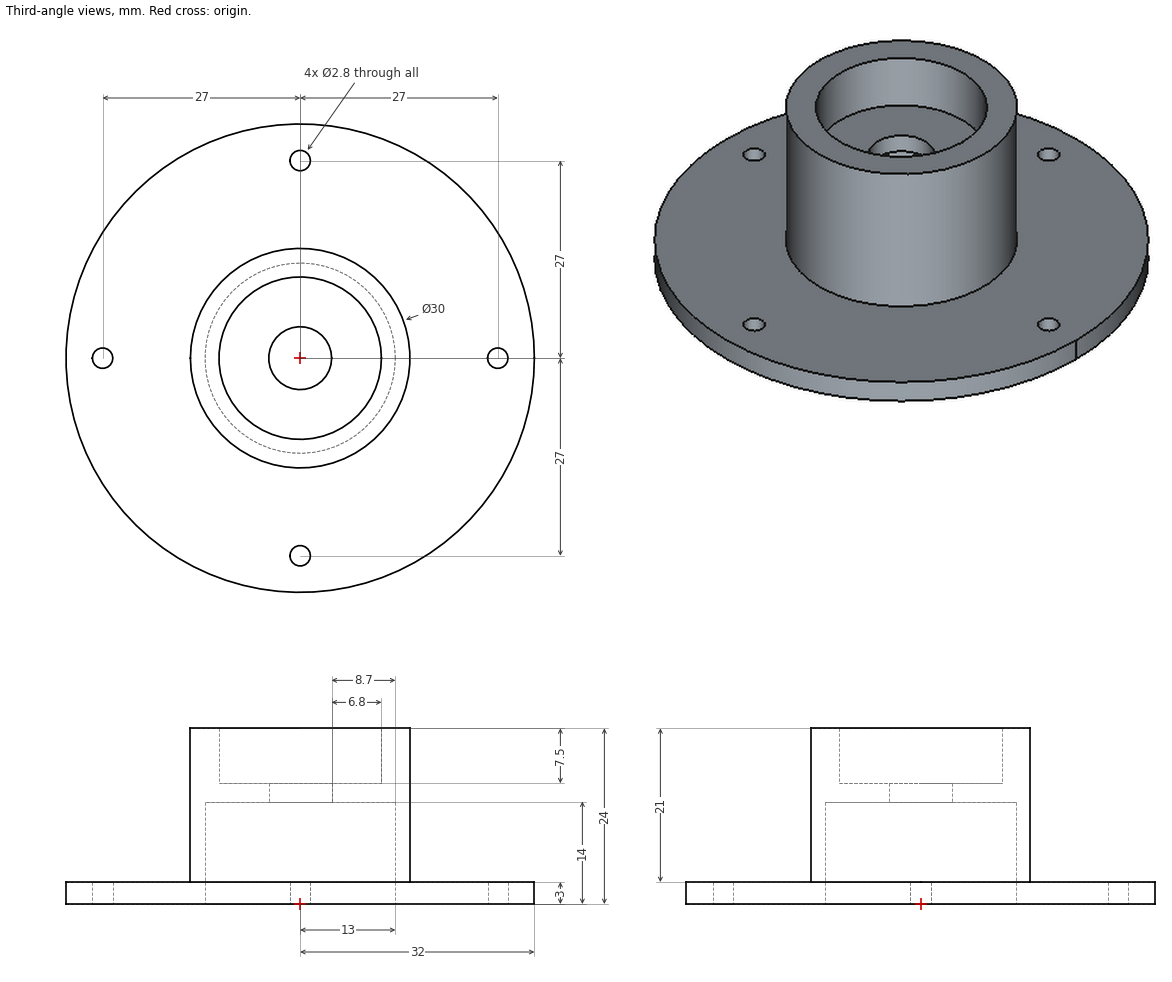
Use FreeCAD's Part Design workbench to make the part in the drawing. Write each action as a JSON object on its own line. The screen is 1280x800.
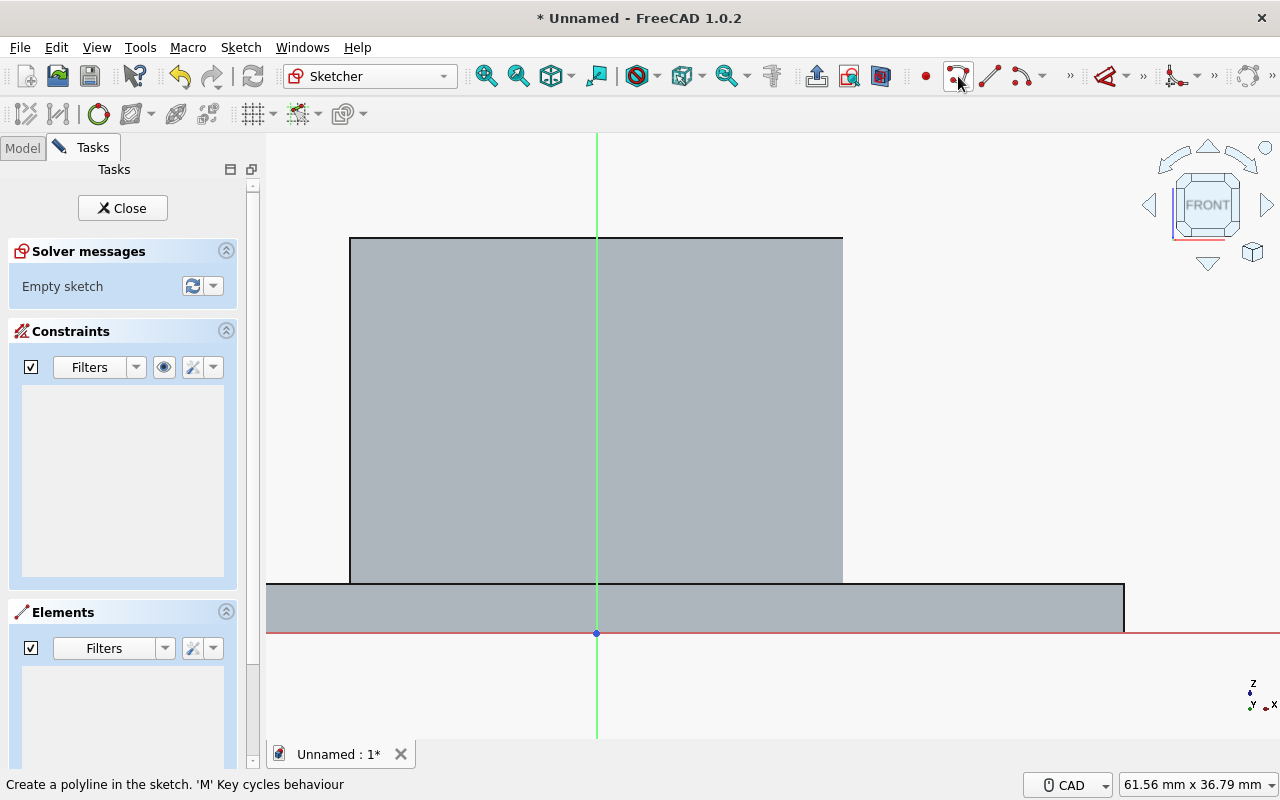
{"action": "left_click", "coordinate": [597, 633]}
{"action": "left_click", "coordinate": [606, 238]}
{"action": "left_click", "coordinate": [780, 238]}
{"action": "left_click", "coordinate": [780, 361]}
{"action": "left_click", "coordinate": [668, 361]}
{"action": "left_click", "coordinate": [668, 402]}
{"action": "left_click", "coordinate": [811, 402]}
{"action": "left_click", "coordinate": [811, 624]}
{"action": "left_click", "coordinate": [597, 633]}
{"action": "key", "text": "Escape"}
{"action": "key", "text": "Escape"}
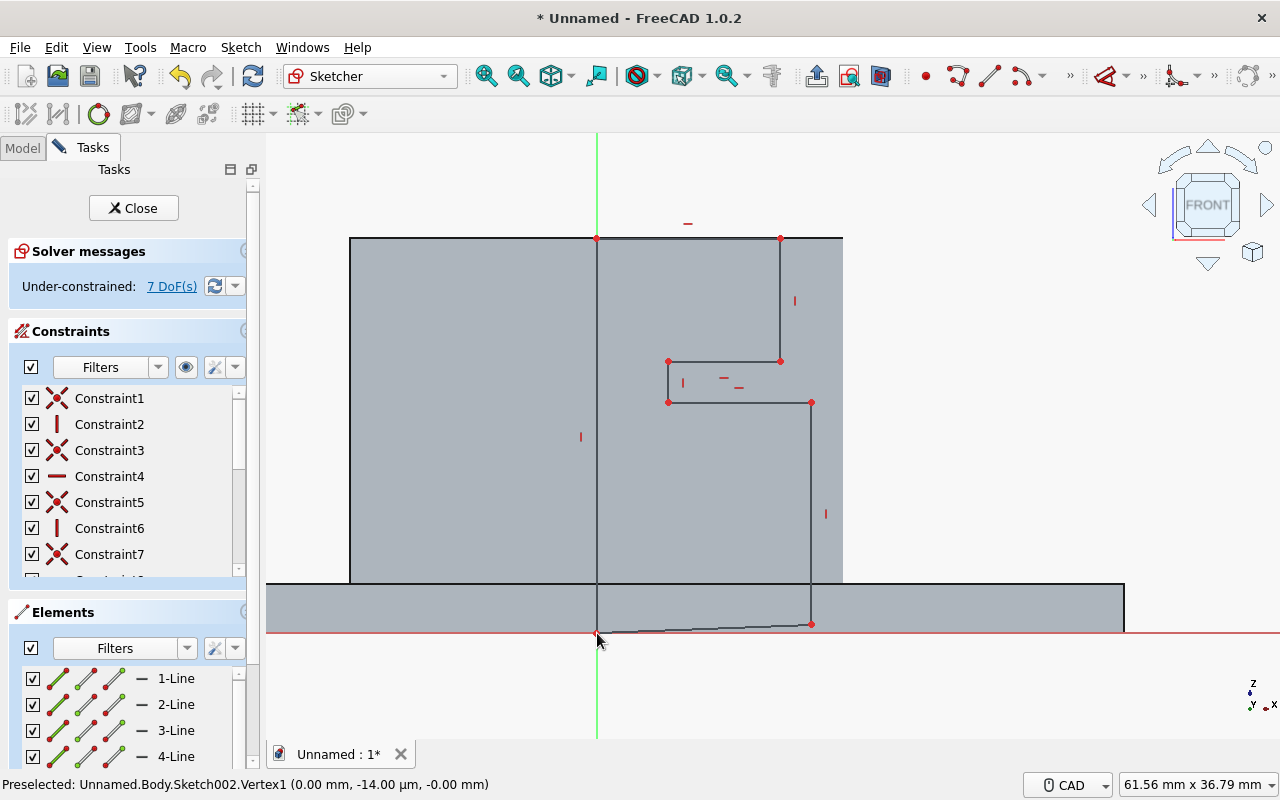
{"action": "left_click", "coordinate": [661, 631]}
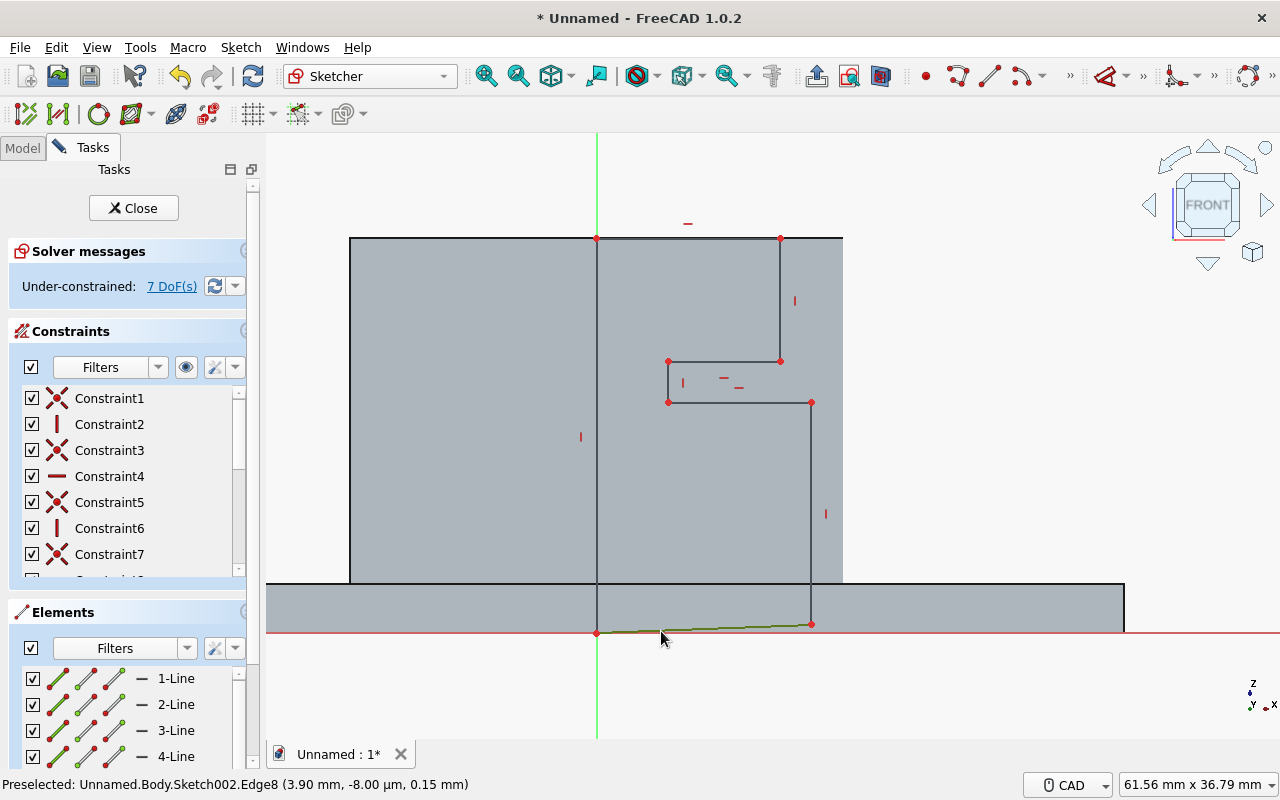
{"action": "key", "text": "h"}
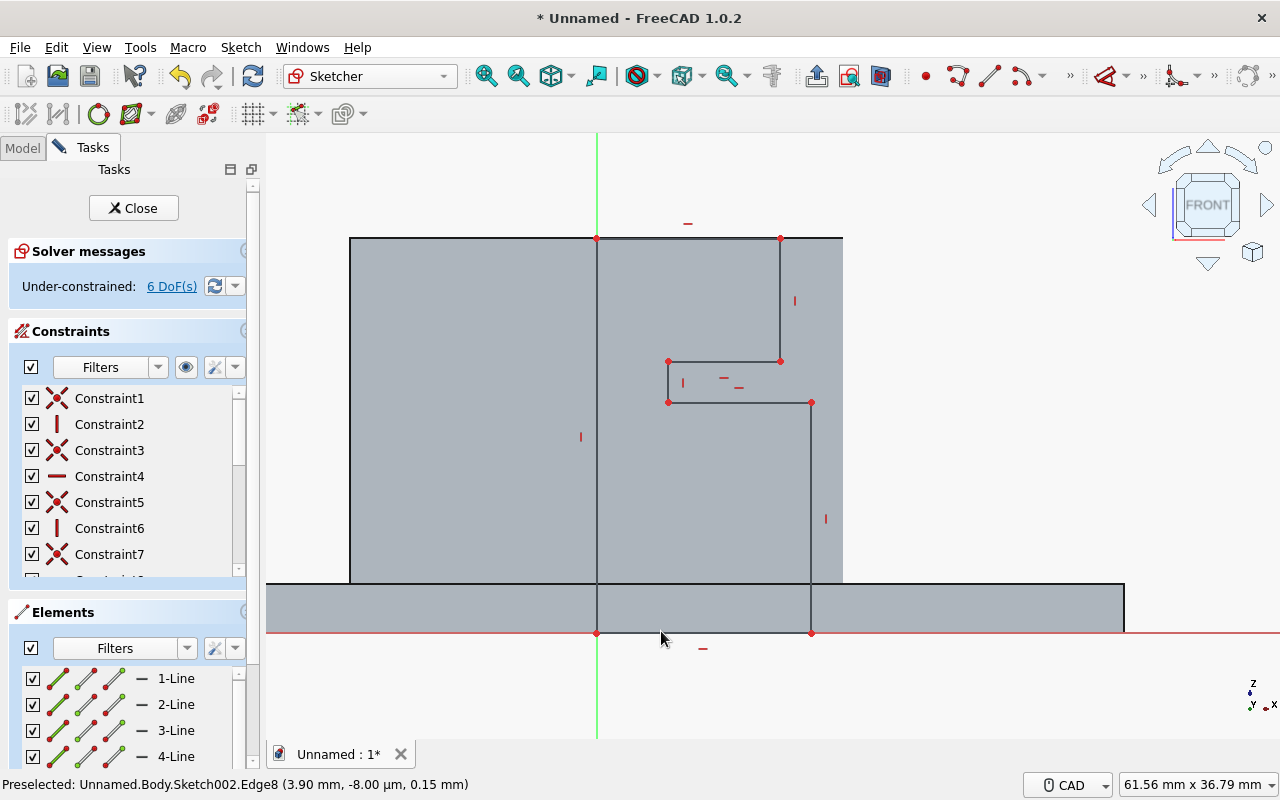
{"action": "key", "text": "d"}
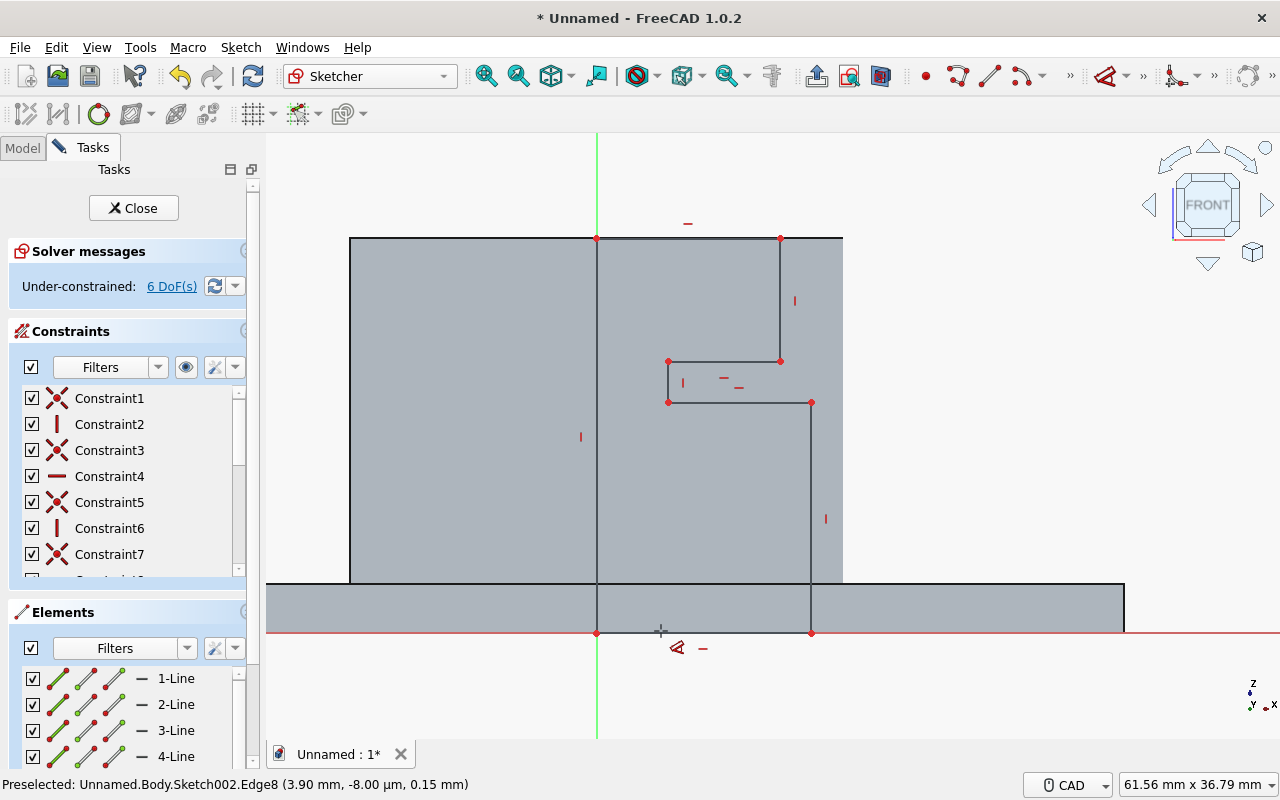
{"action": "left_click", "coordinate": [597, 515]}
{"action": "left_click", "coordinate": [563, 436]}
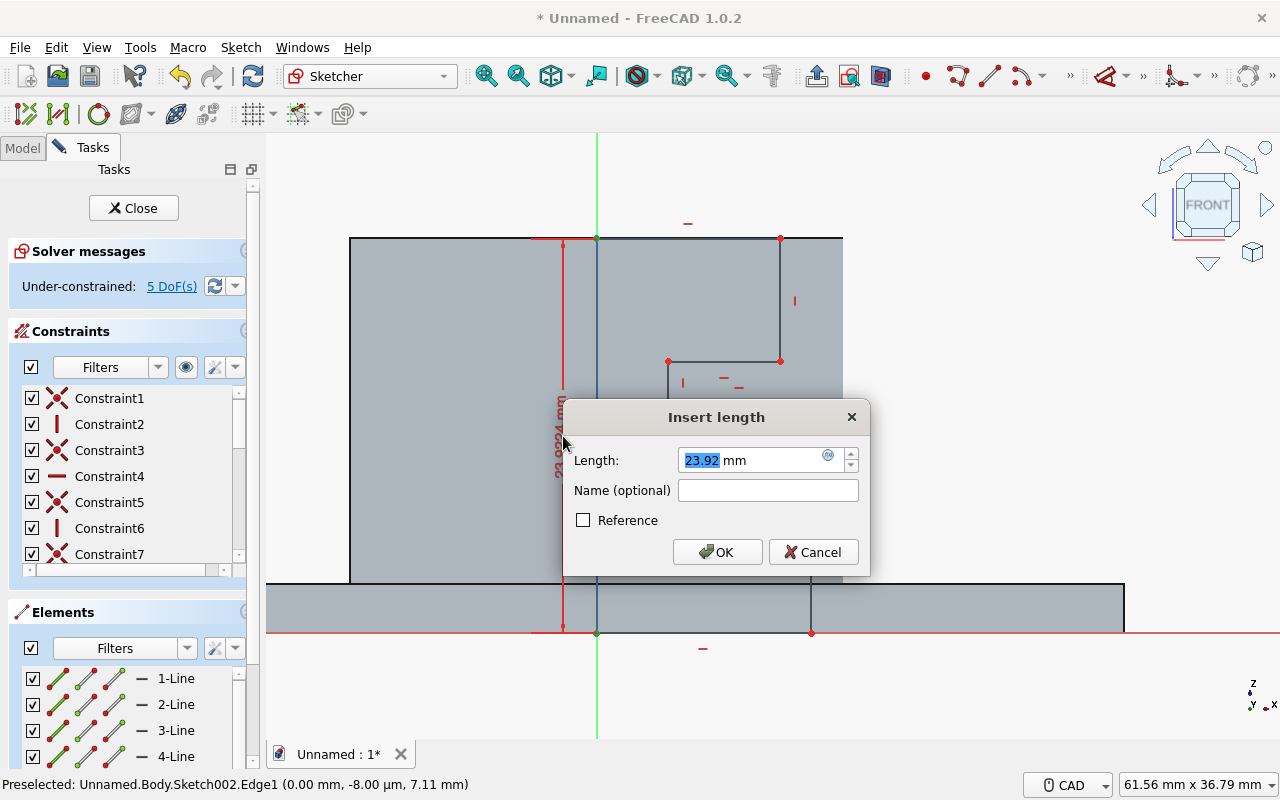
{"action": "type", "text": "24"}
{"action": "key", "text": "Return"}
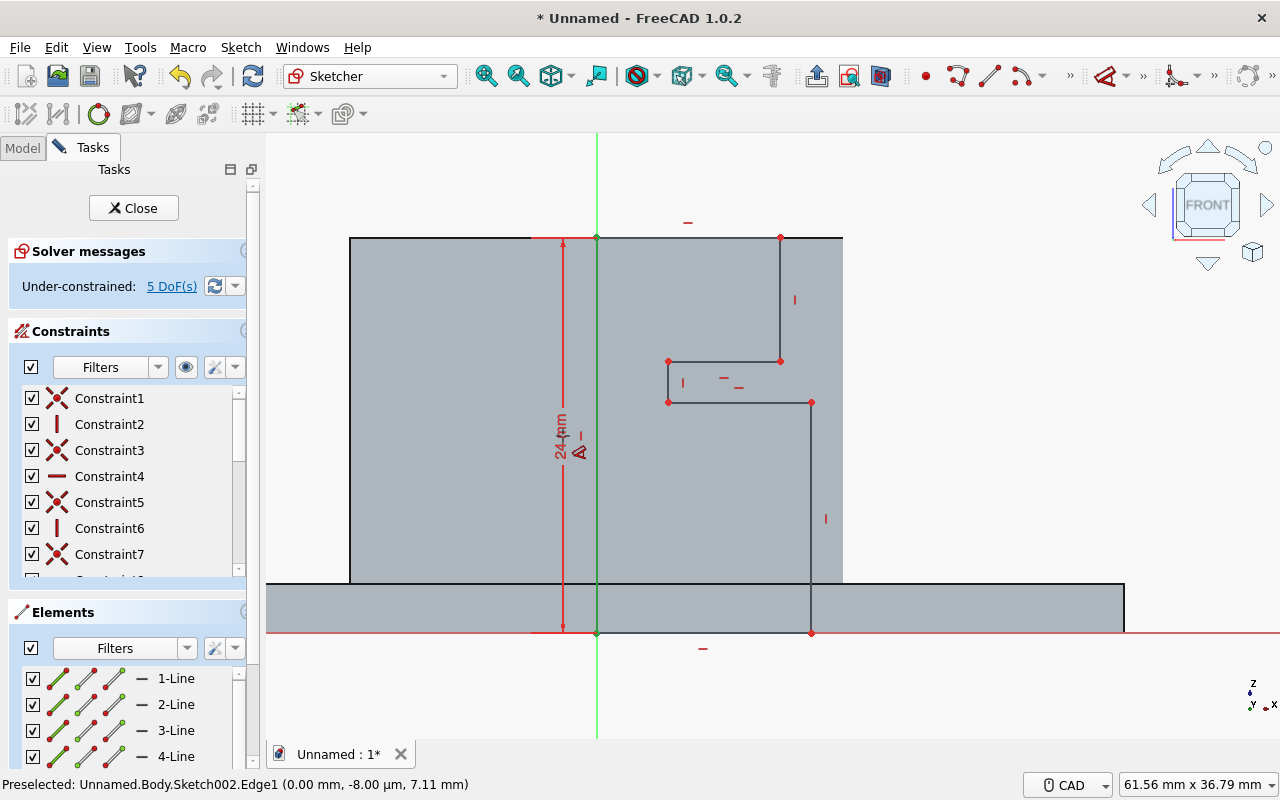
{"action": "left_click", "coordinate": [811, 472]}
{"action": "left_click", "coordinate": [845, 518]}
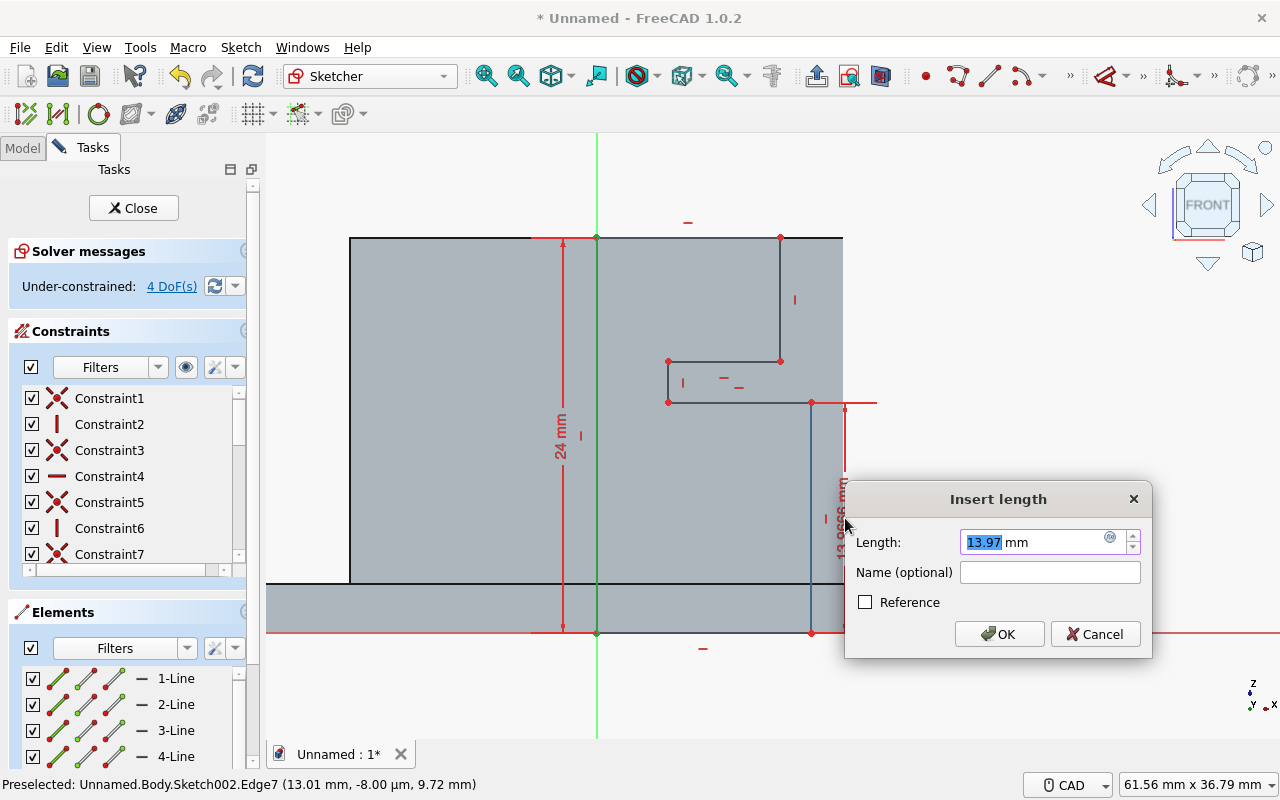
{"action": "type", "text": "14"}
{"action": "key", "text": "Return"}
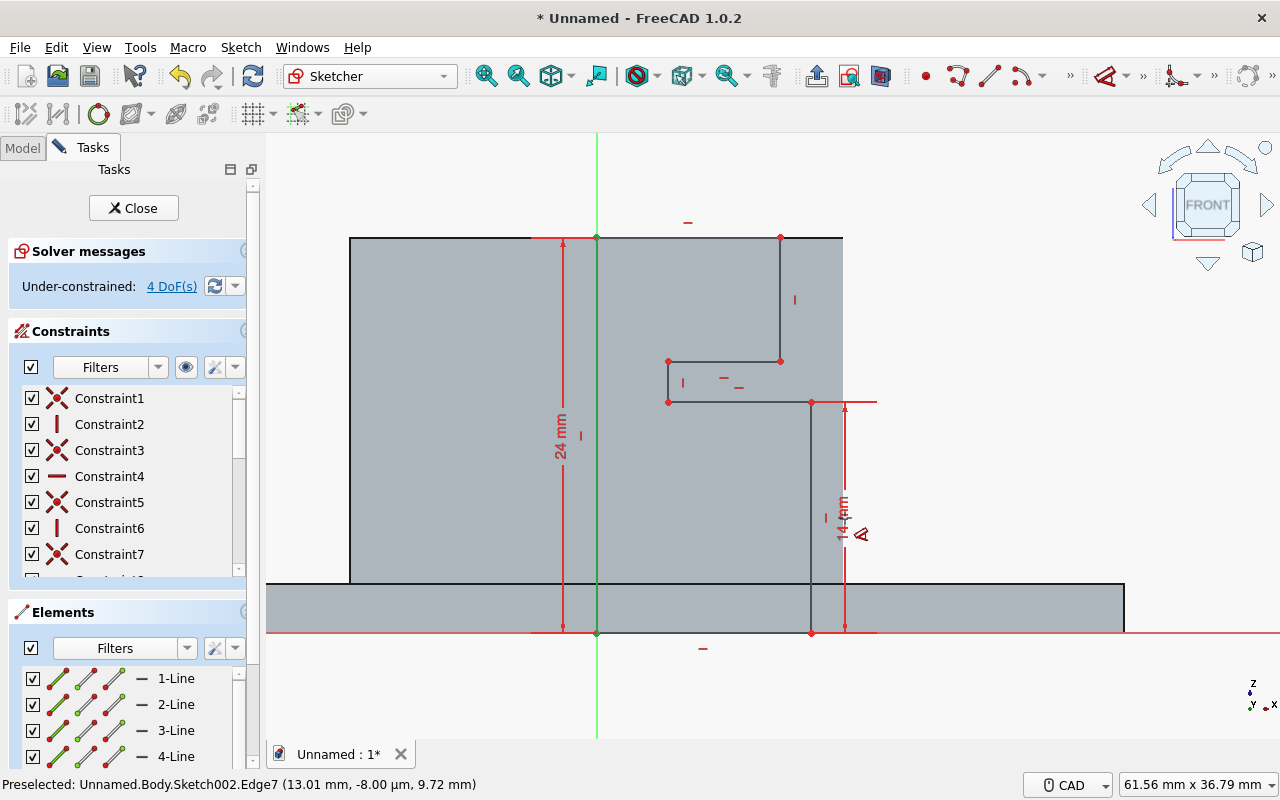
{"action": "left_click", "coordinate": [747, 633]}
{"action": "left_click", "coordinate": [704, 667]}